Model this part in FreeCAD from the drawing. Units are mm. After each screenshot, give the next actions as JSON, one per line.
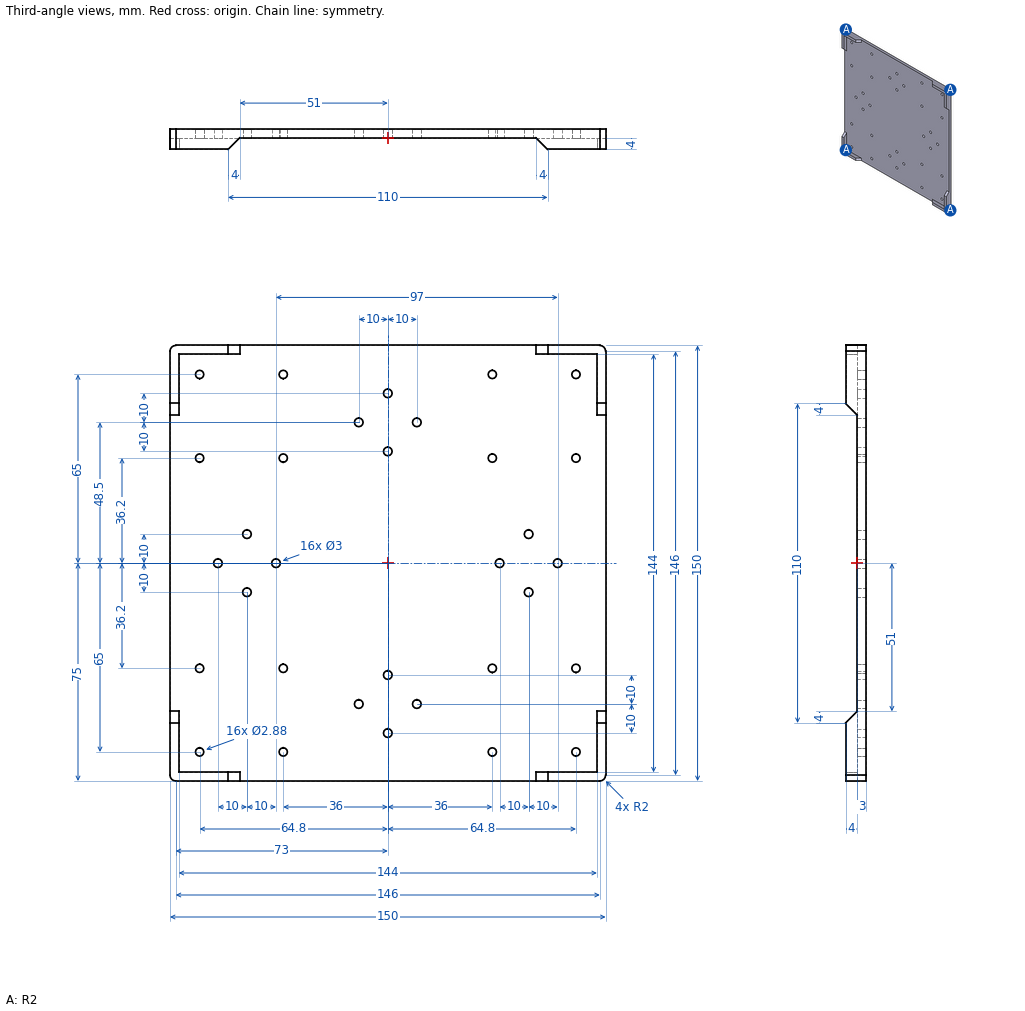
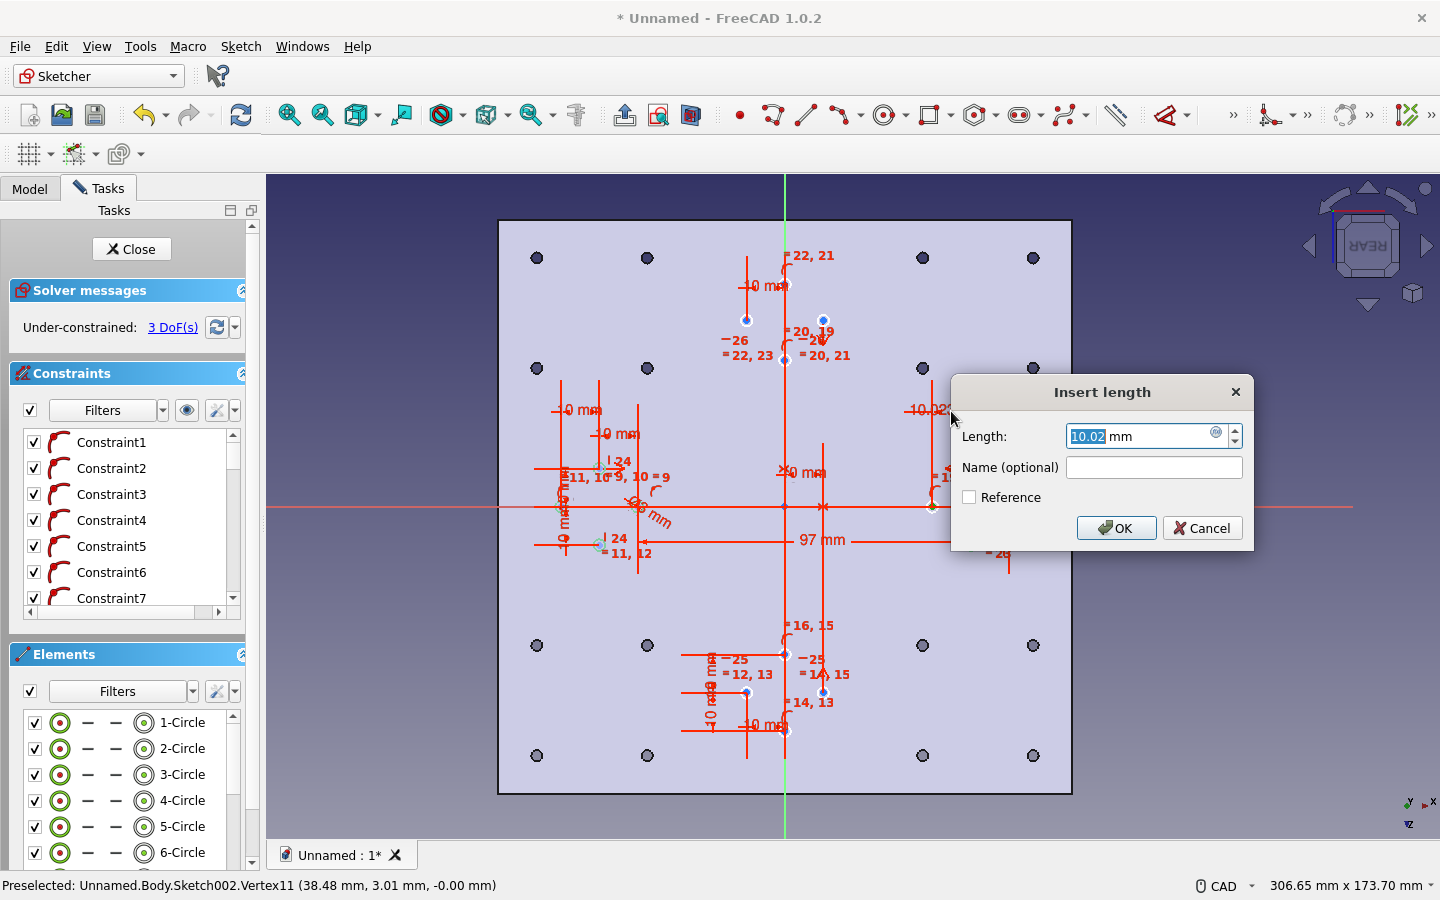
{"action": "type", "text": "10"}
{"action": "key", "text": "Return"}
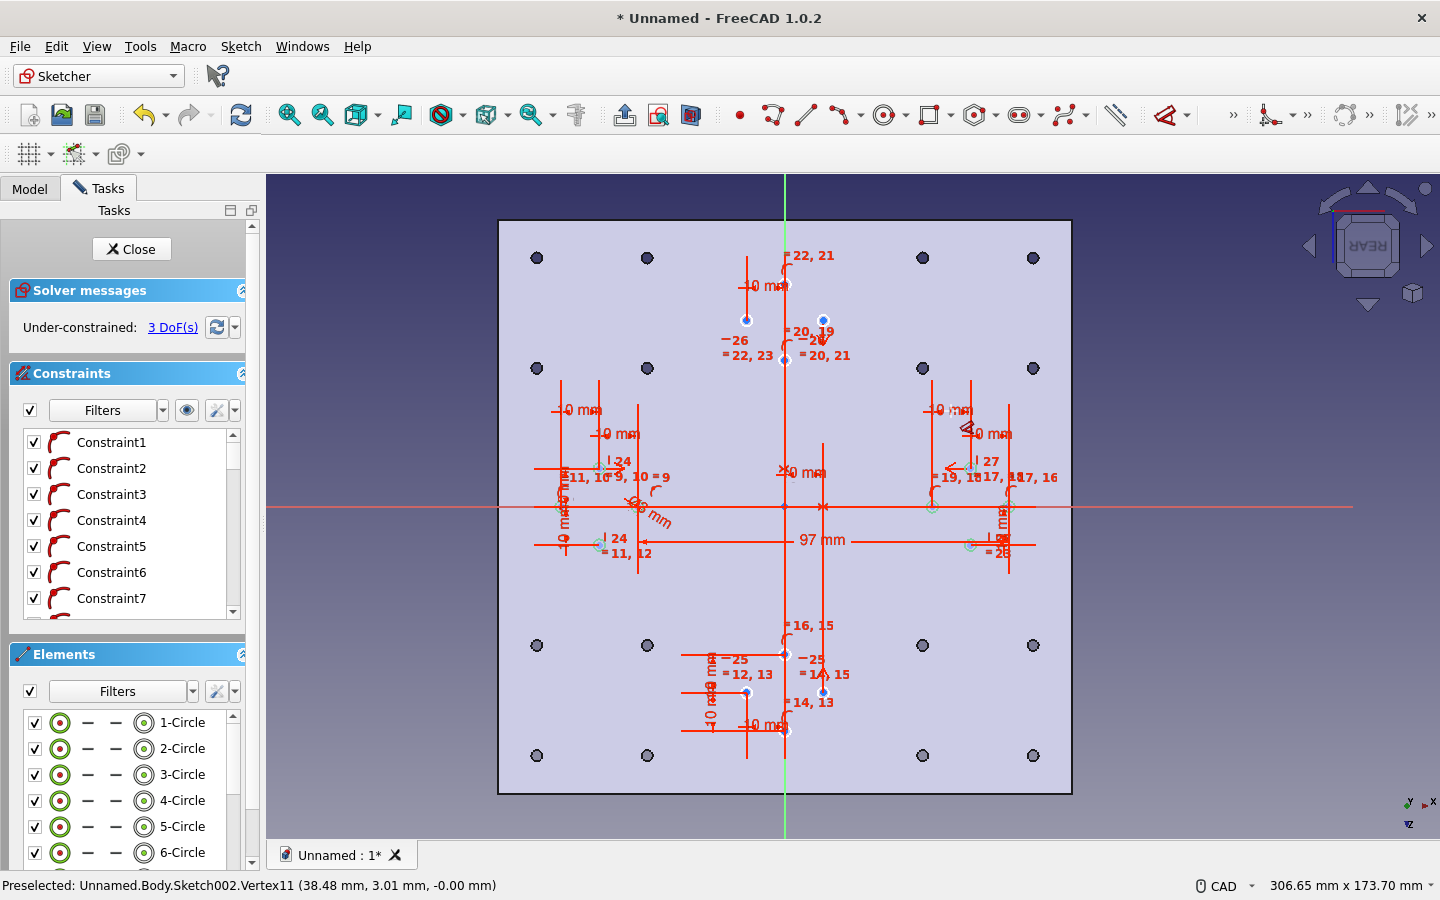
{"action": "left_click", "coordinate": [785, 360]}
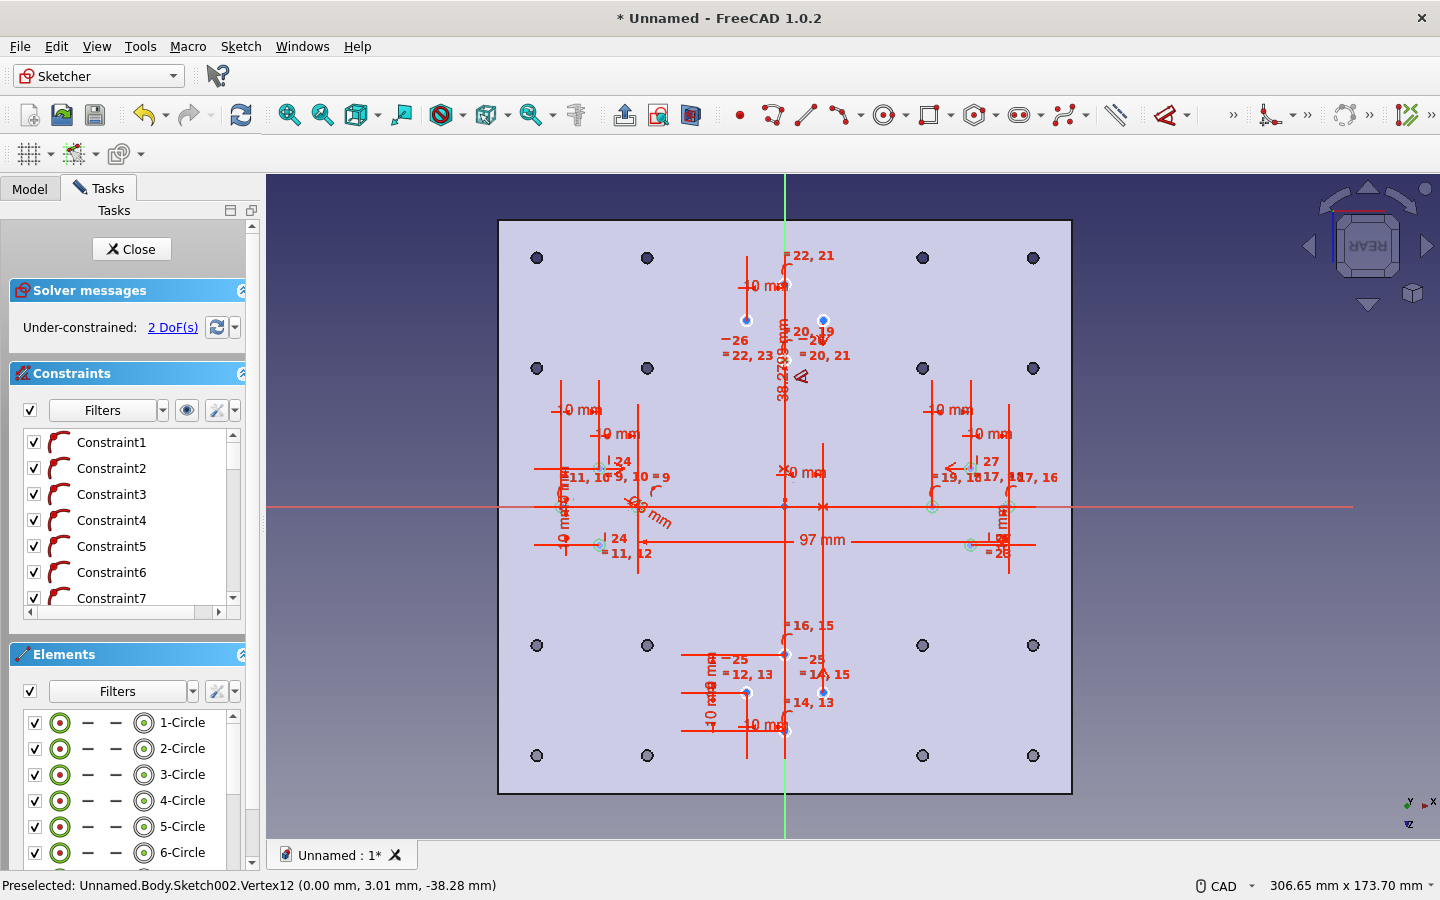
{"action": "left_click", "coordinate": [823, 321]}
{"action": "left_click", "coordinate": [857, 341]}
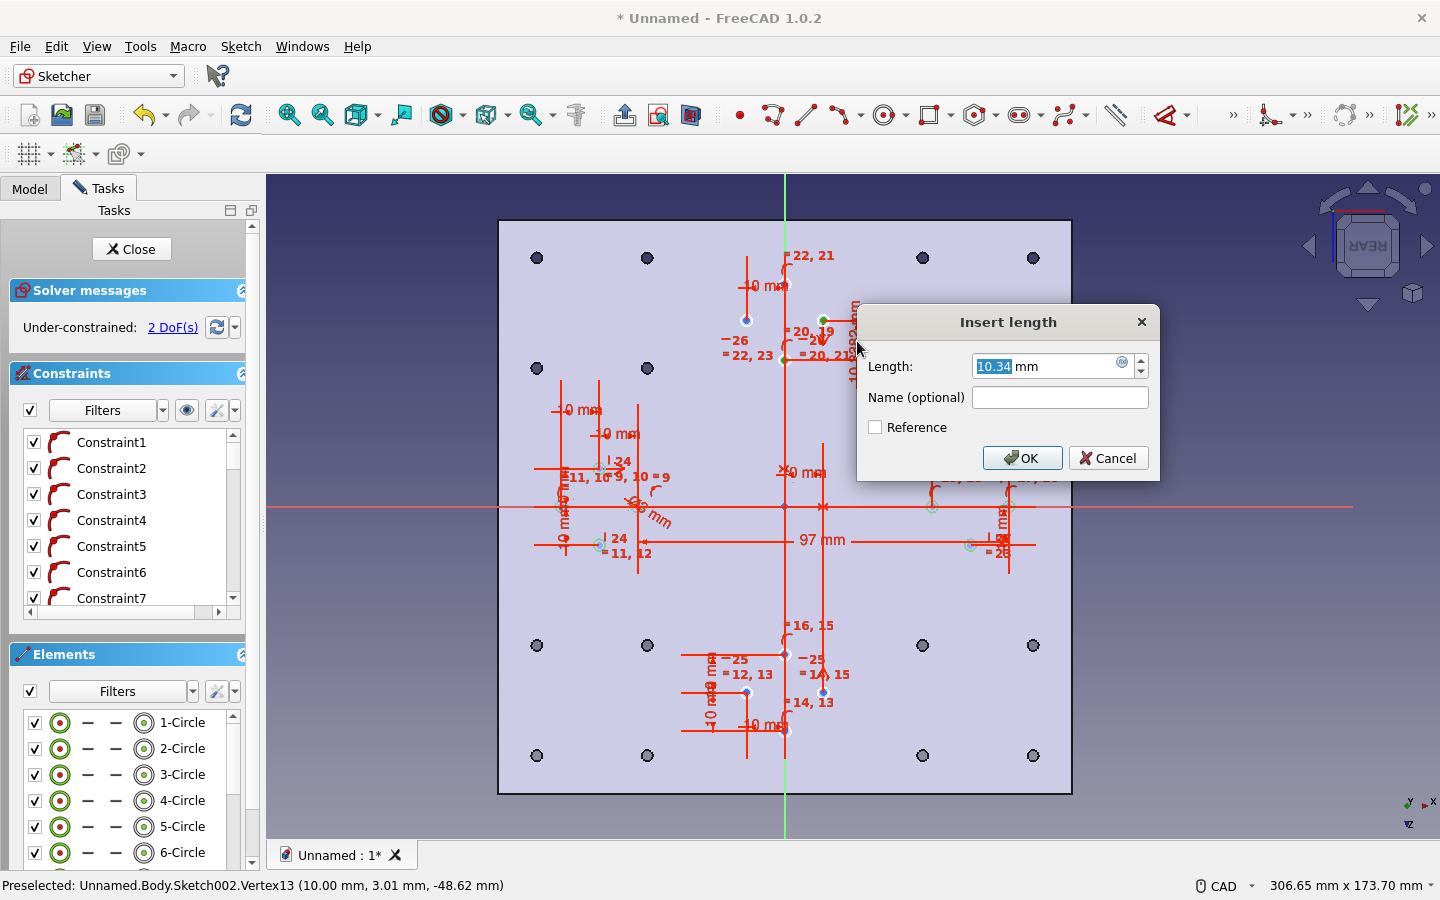
{"action": "type", "text": "10"}
{"action": "key", "text": "Return"}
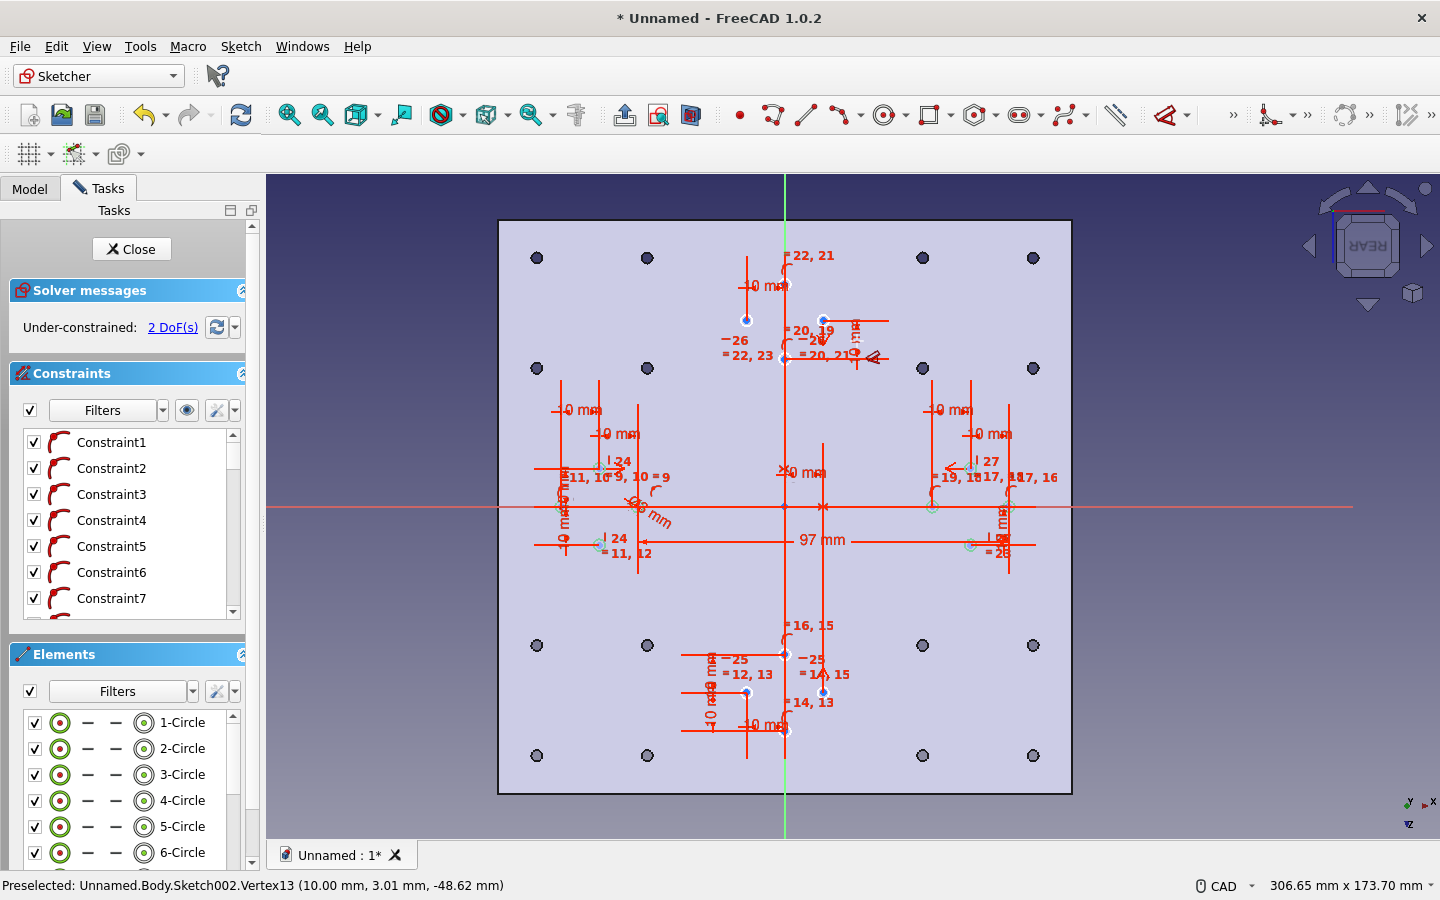
{"action": "left_click", "coordinate": [823, 321]}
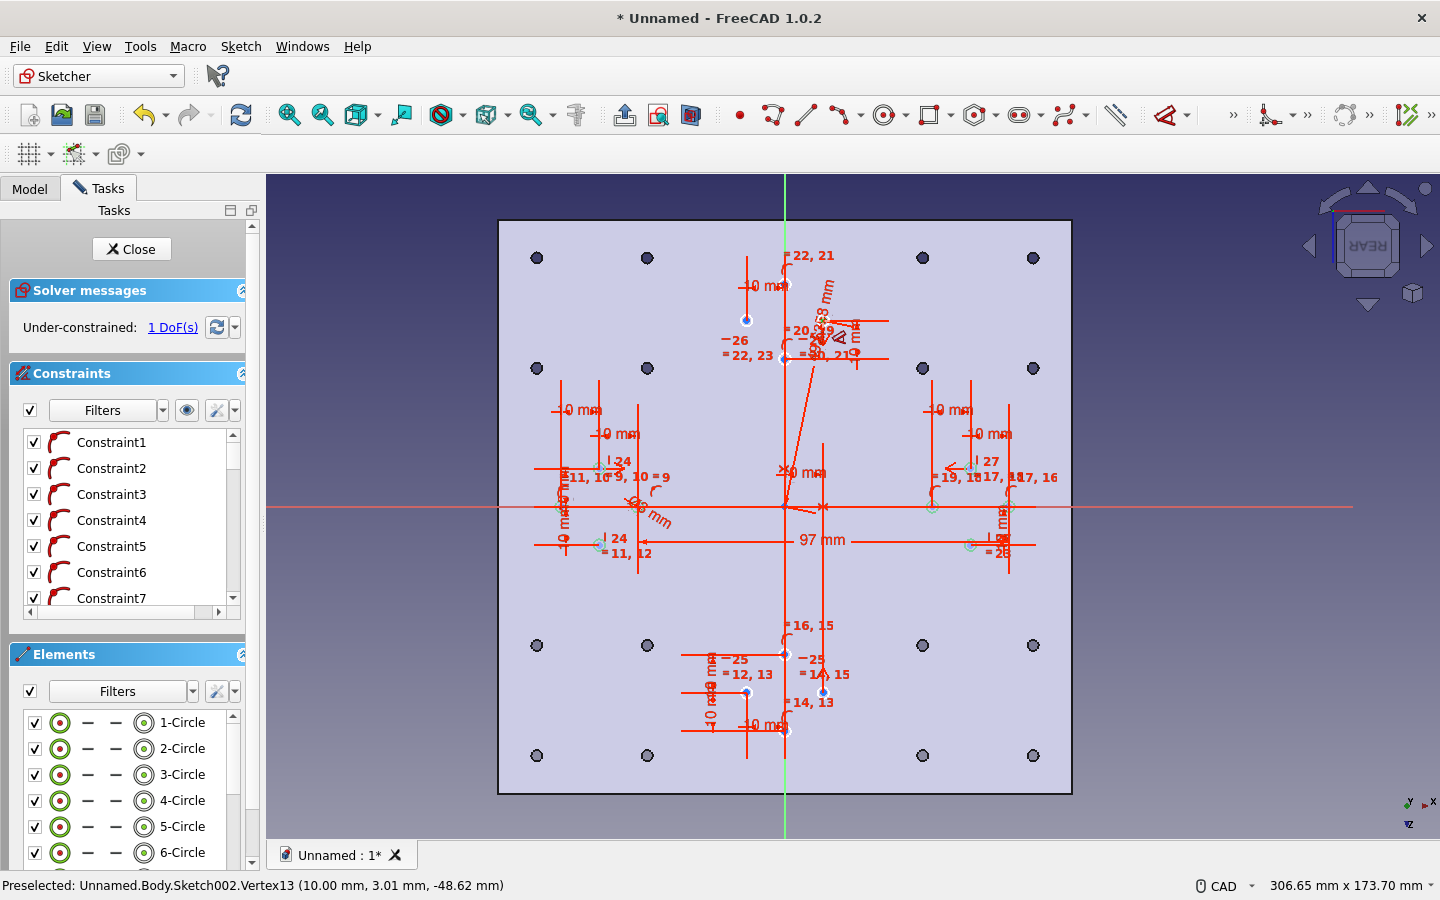
{"action": "left_click", "coordinate": [785, 284]}
{"action": "left_click", "coordinate": [857, 303]}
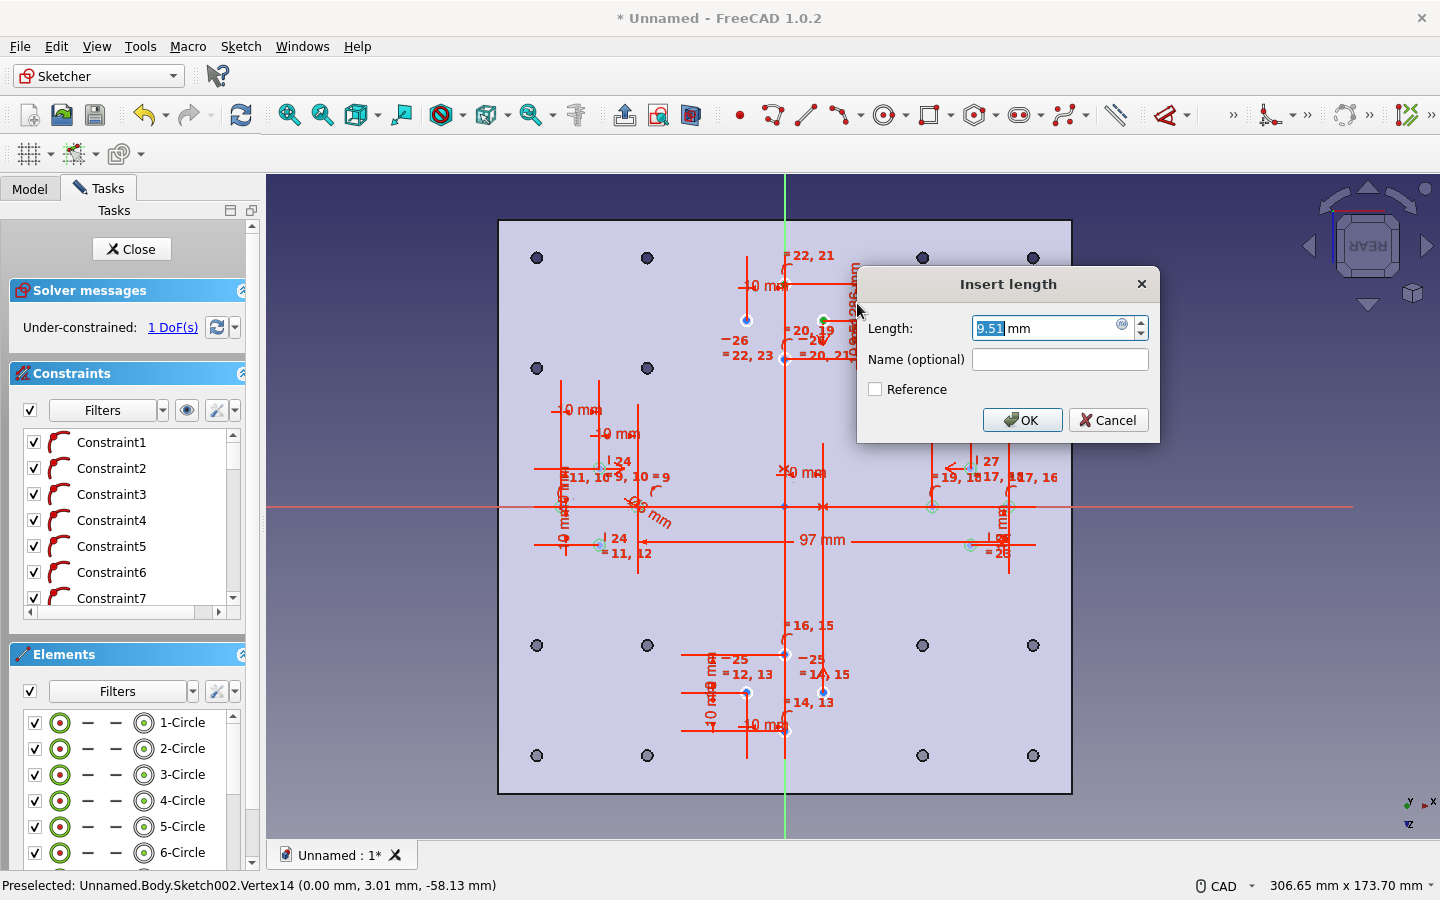
{"action": "type", "text": "10"}
{"action": "key", "text": "Return"}